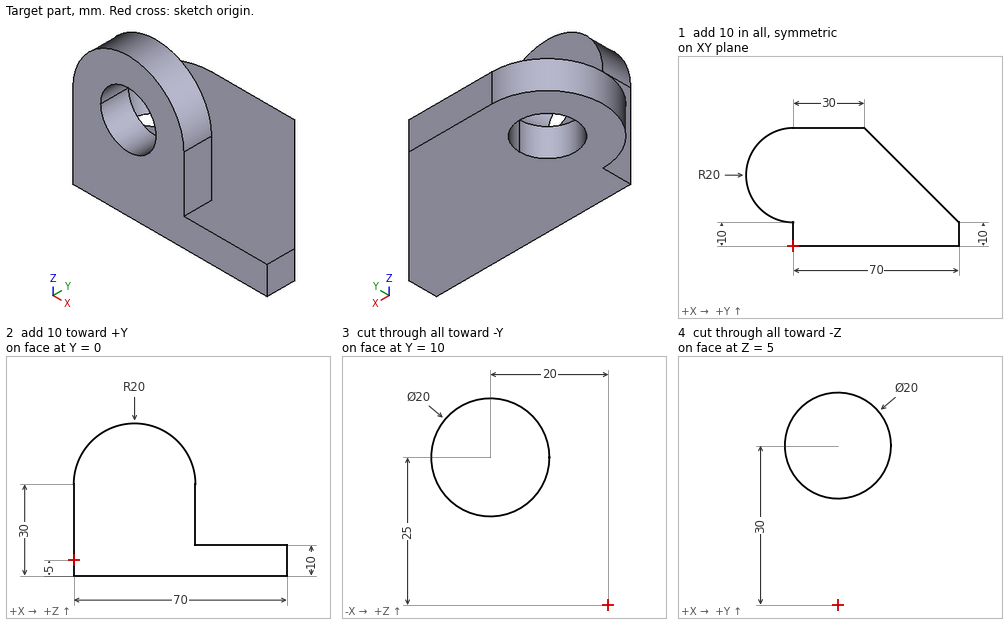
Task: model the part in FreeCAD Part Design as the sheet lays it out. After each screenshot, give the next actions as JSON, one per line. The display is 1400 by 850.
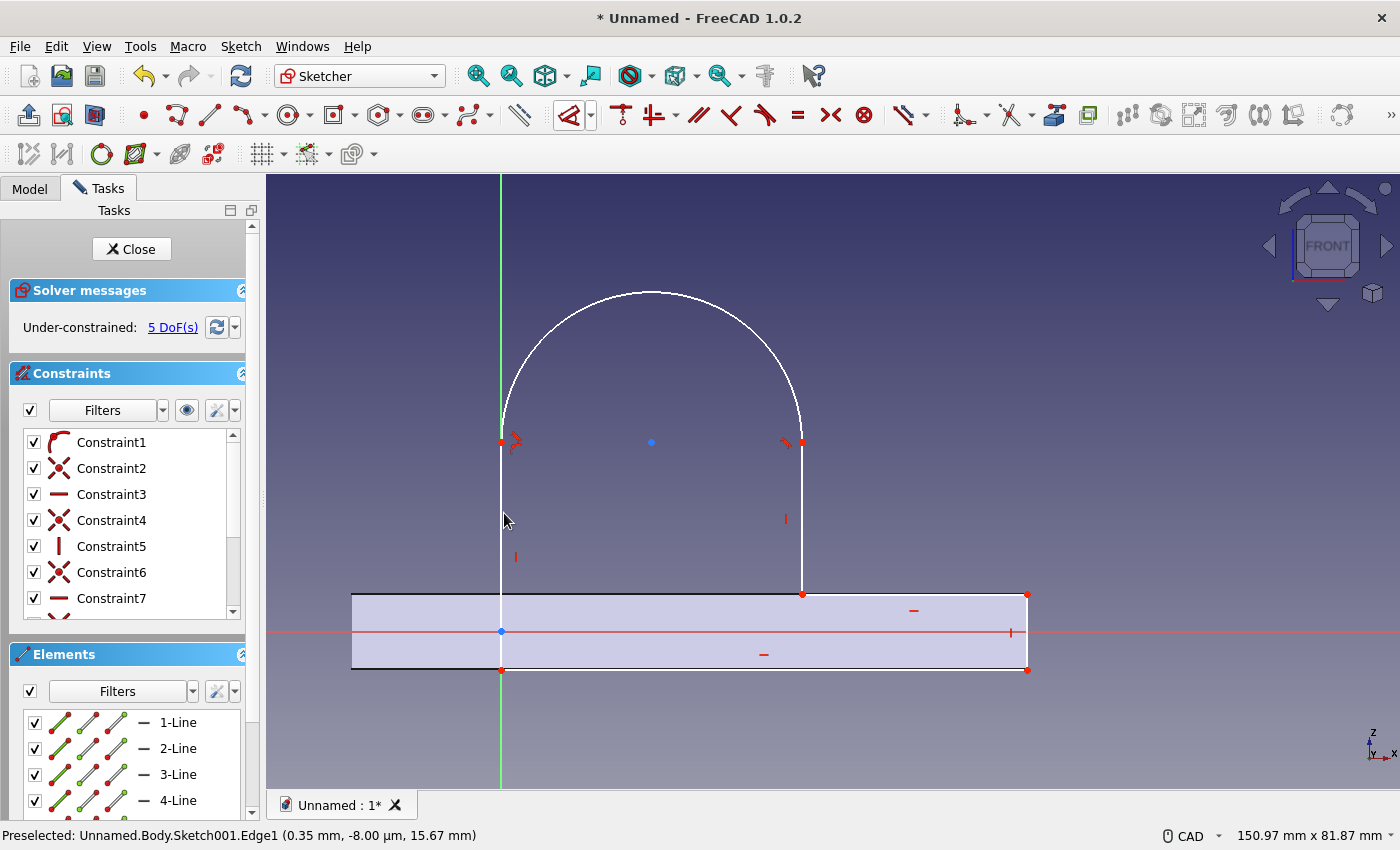
{"action": "left_click", "coordinate": [740, 321]}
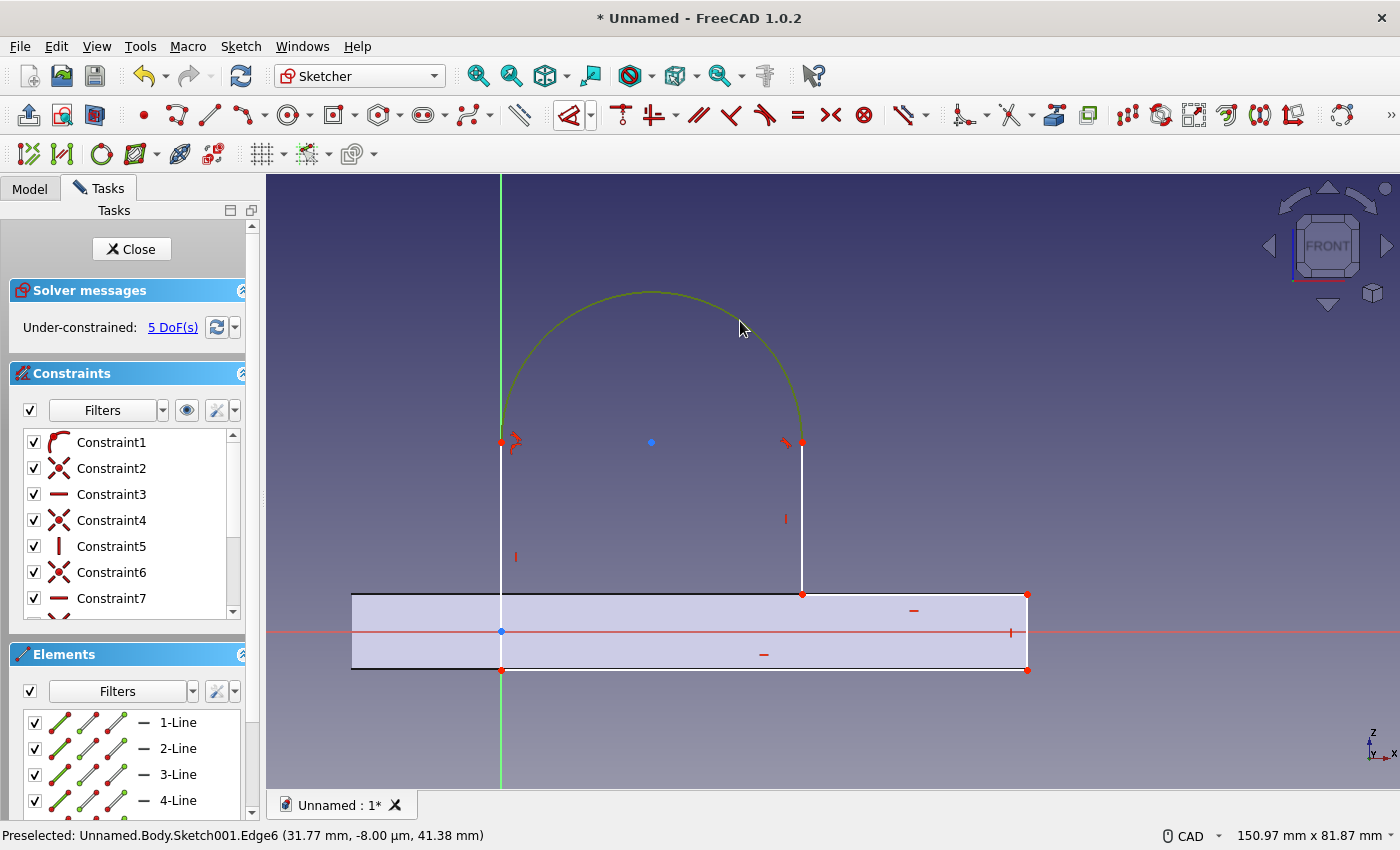
{"action": "key", "text": "k r"}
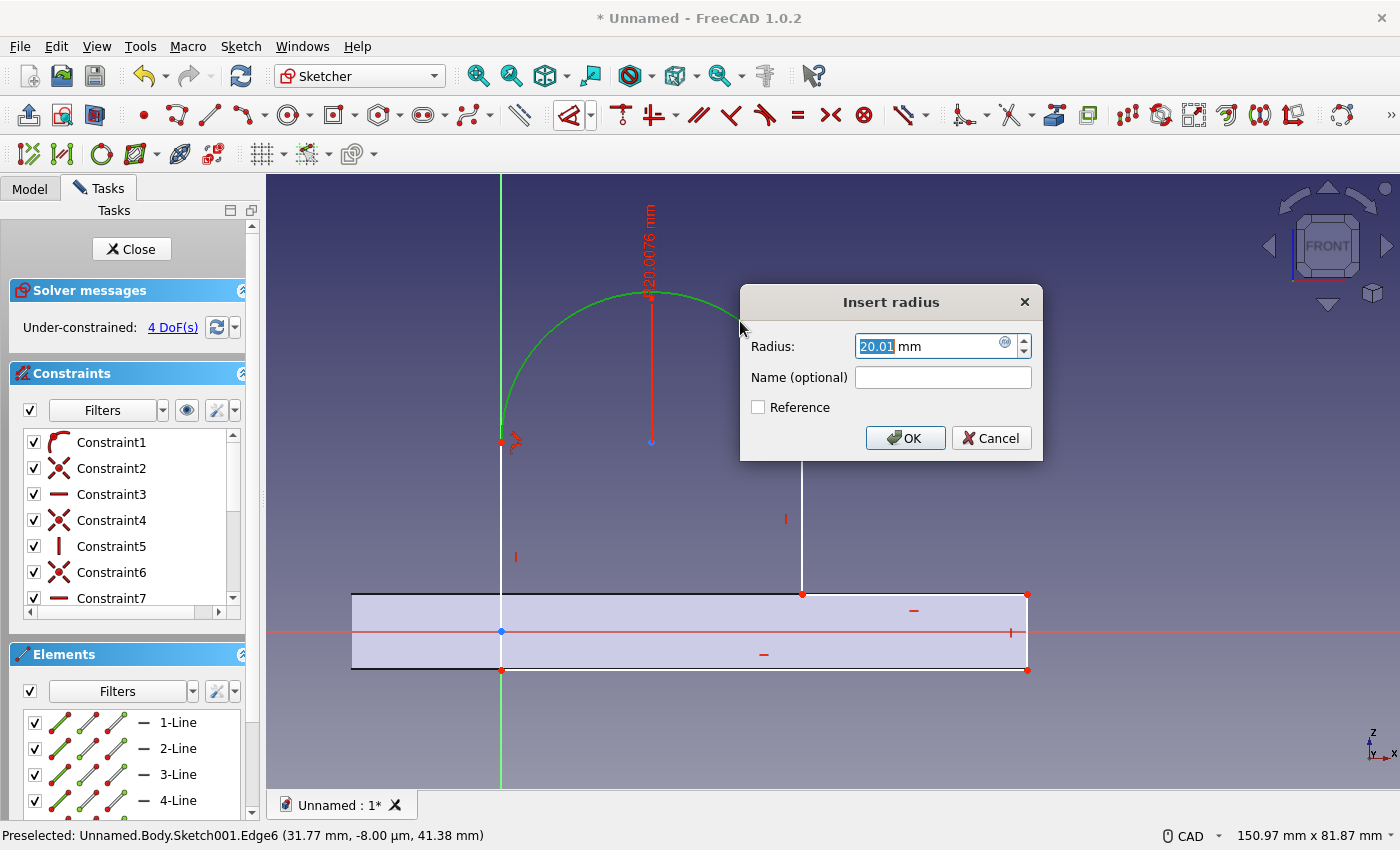
{"action": "type", "text": "20"}
{"action": "key", "text": "Return"}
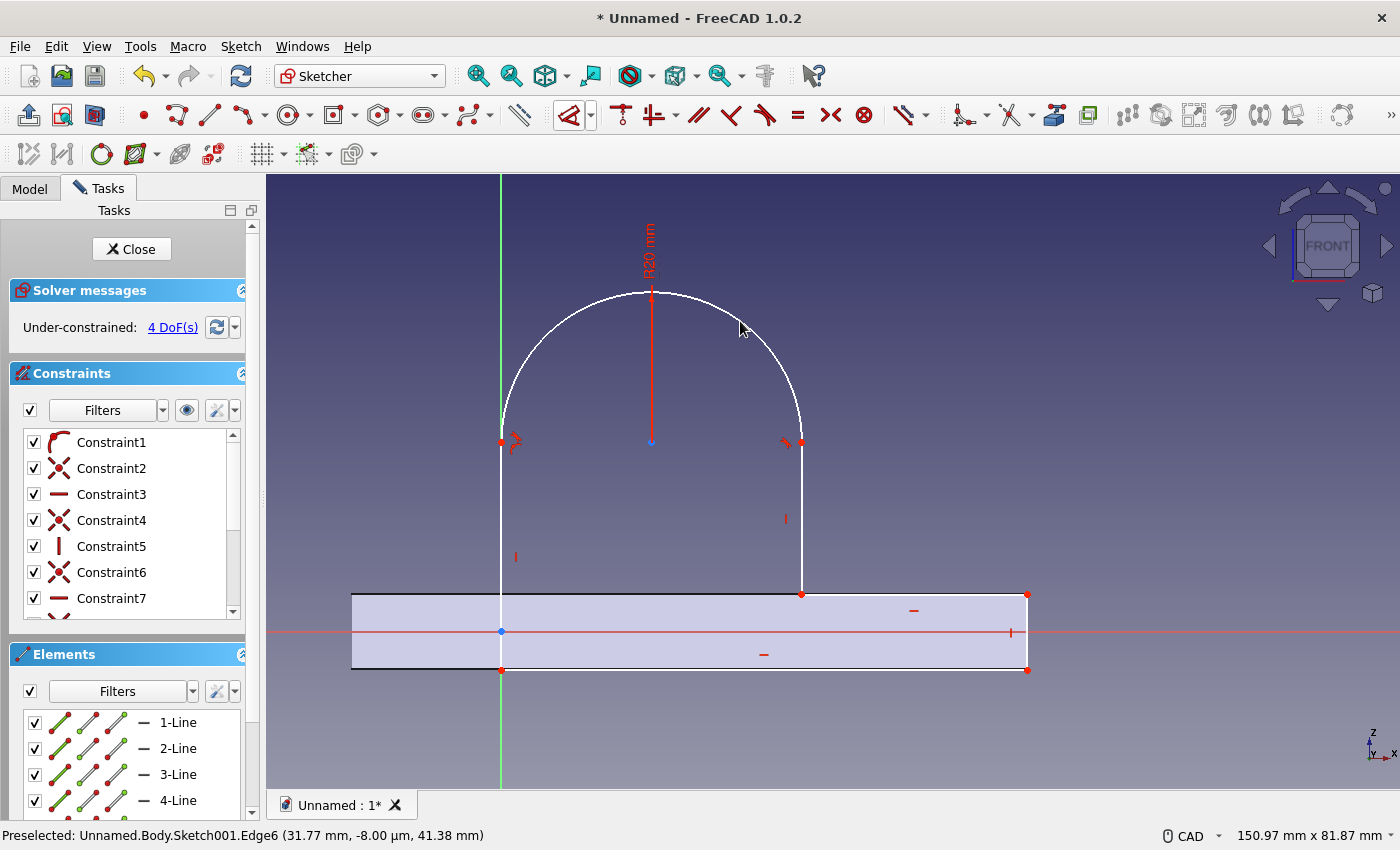
{"action": "left_click", "coordinate": [501, 511]}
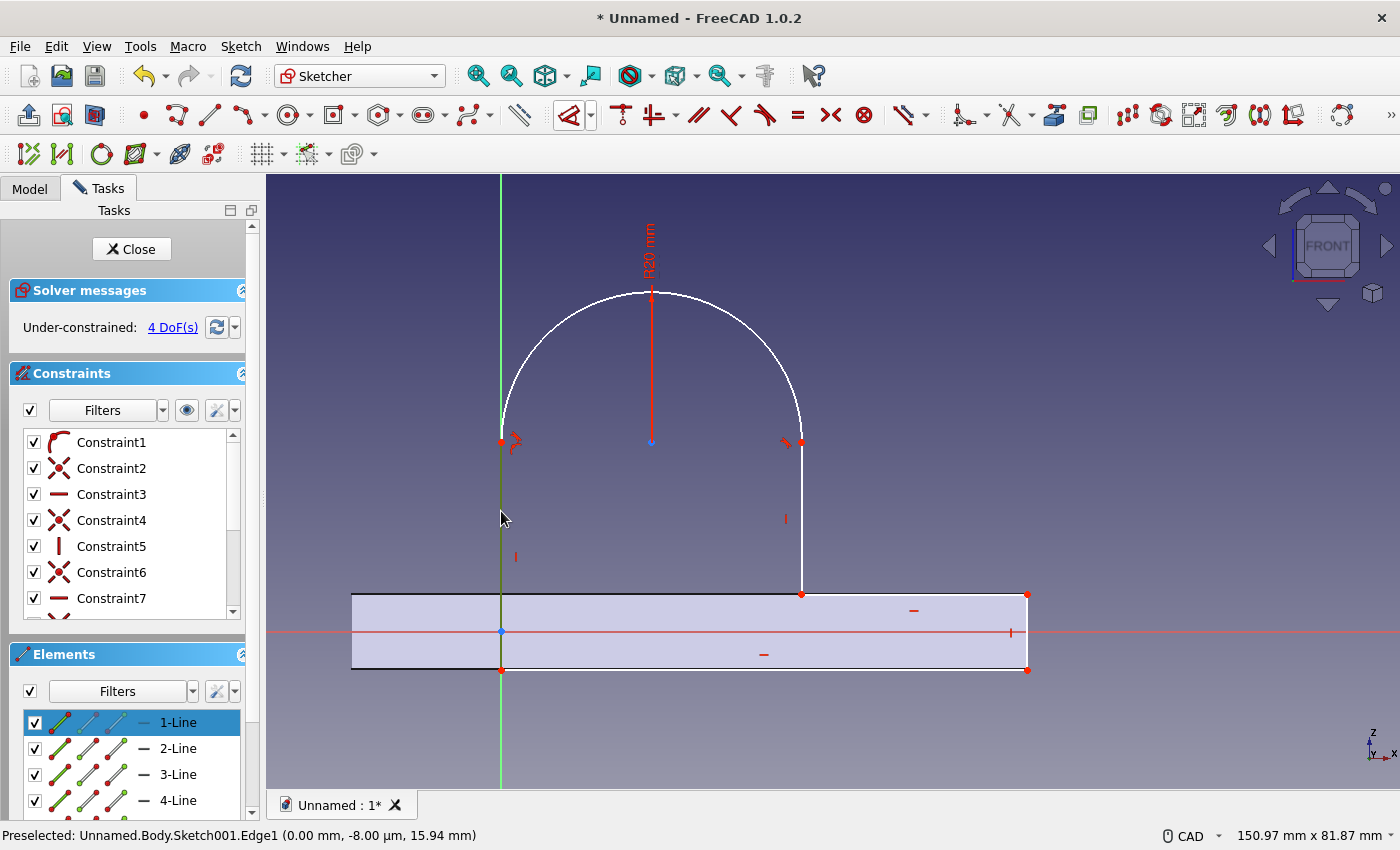
{"action": "key", "text": "i"}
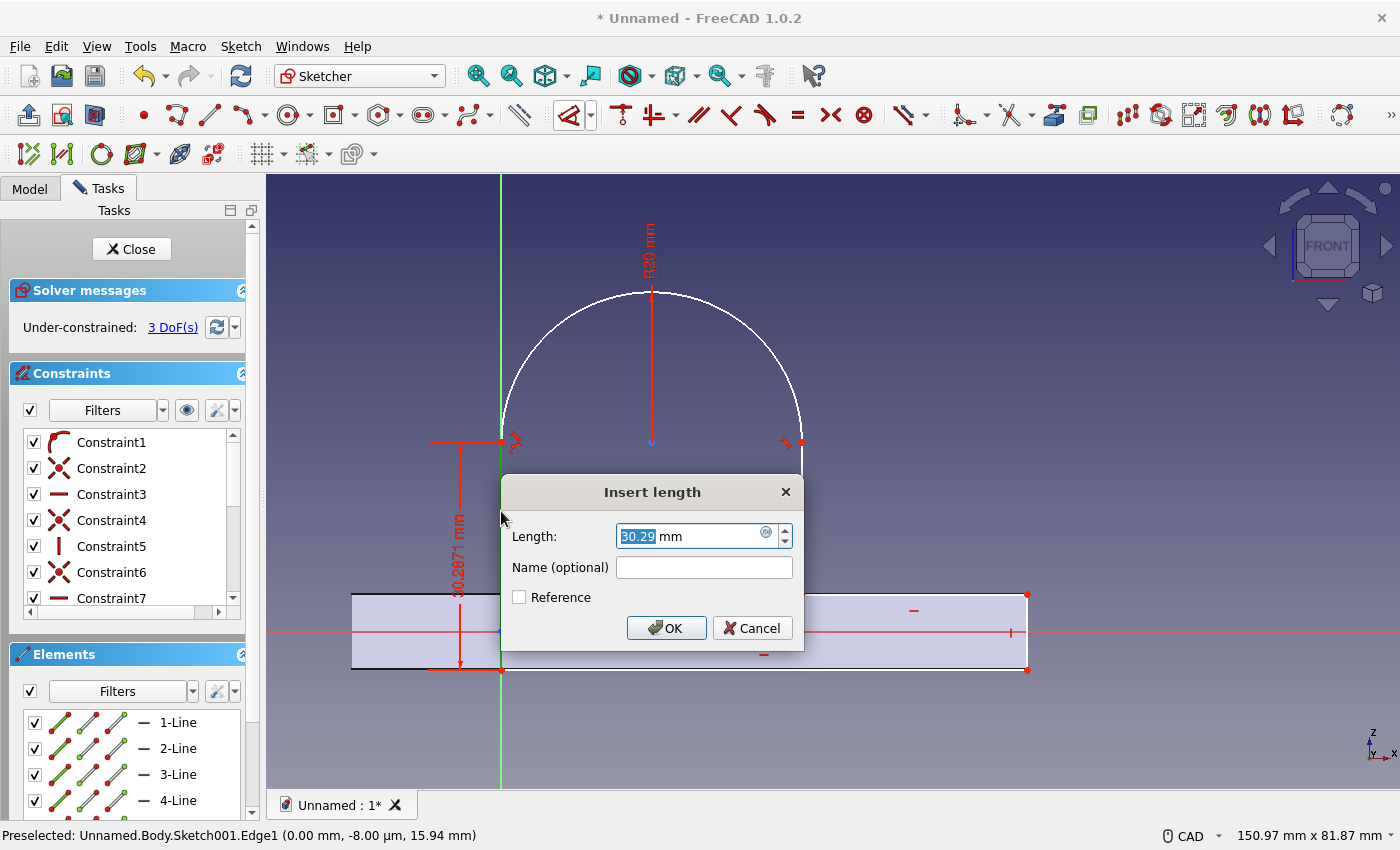
{"action": "type", "text": "30"}
{"action": "key", "text": "Return"}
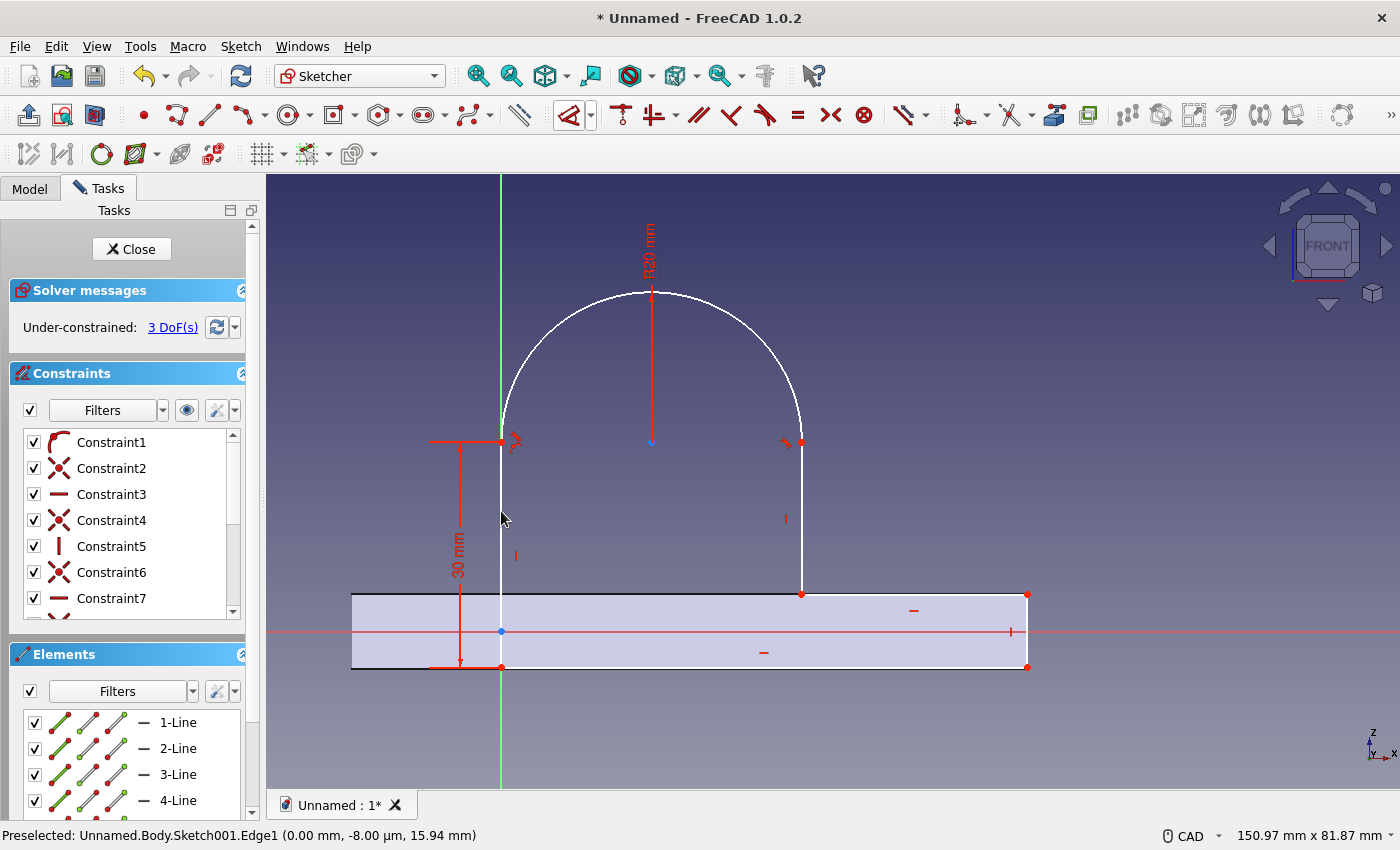
{"action": "left_click", "coordinate": [659, 668]}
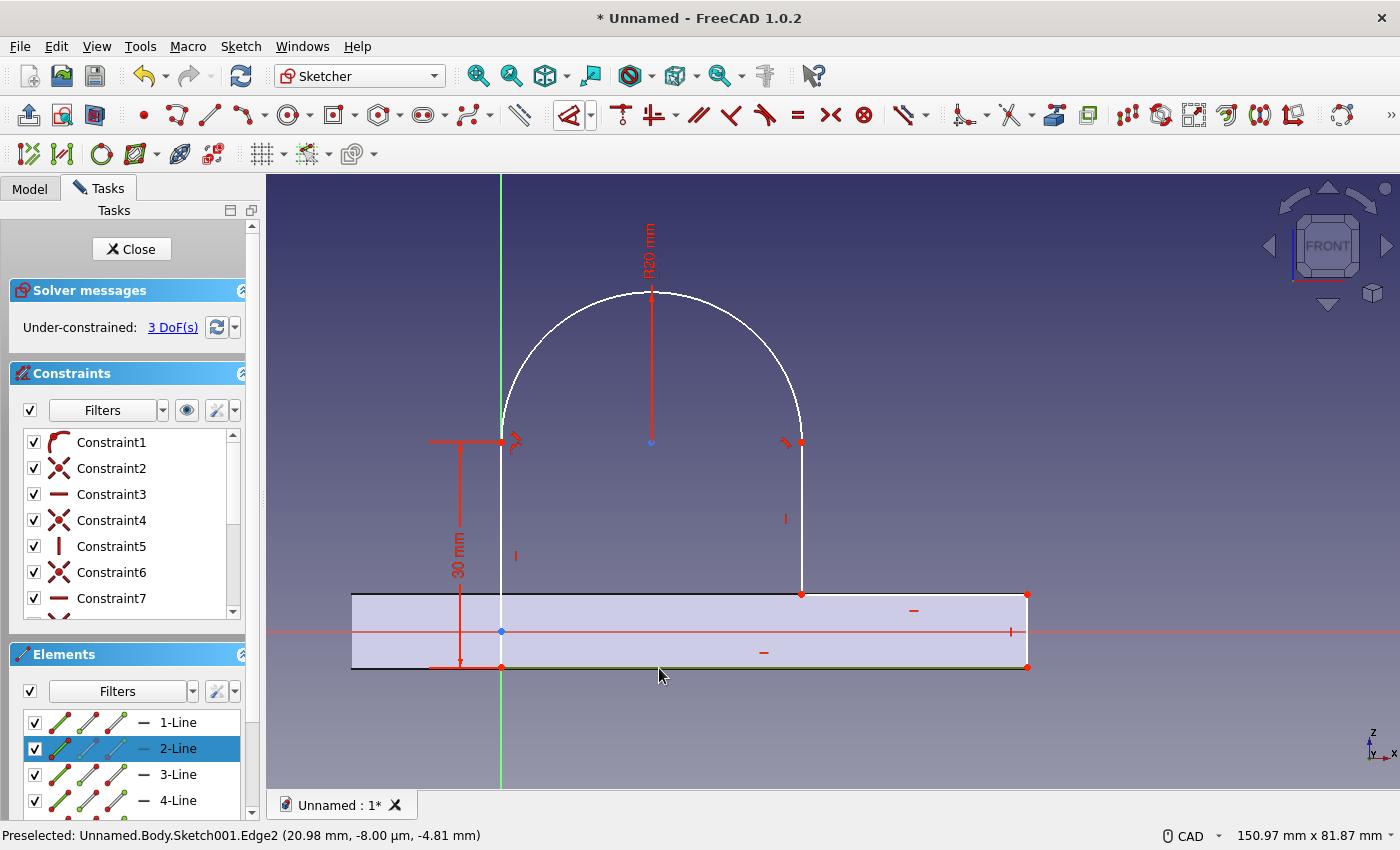
{"action": "key", "text": "l"}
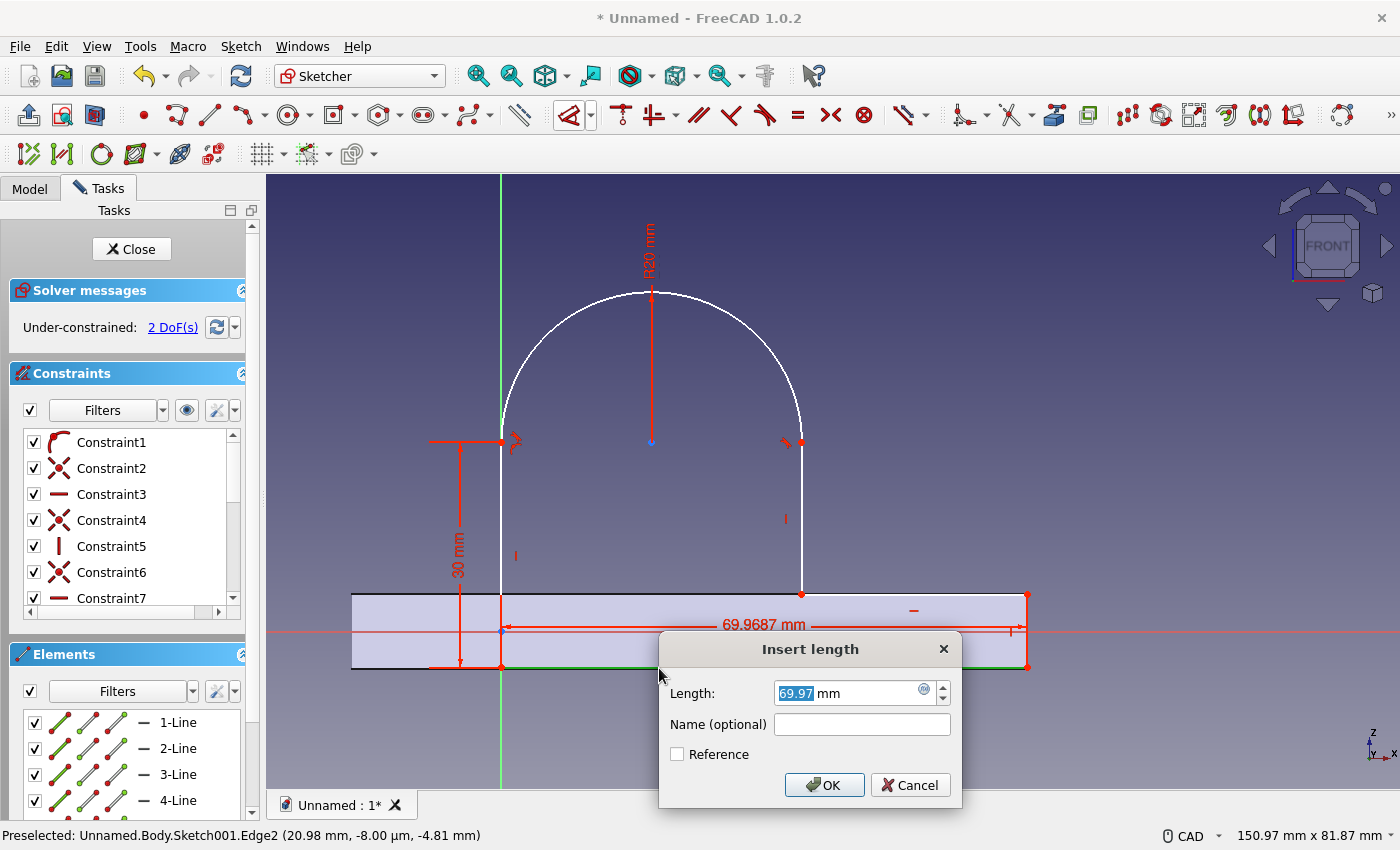
{"action": "type", "text": "70"}
{"action": "key", "text": "Return"}